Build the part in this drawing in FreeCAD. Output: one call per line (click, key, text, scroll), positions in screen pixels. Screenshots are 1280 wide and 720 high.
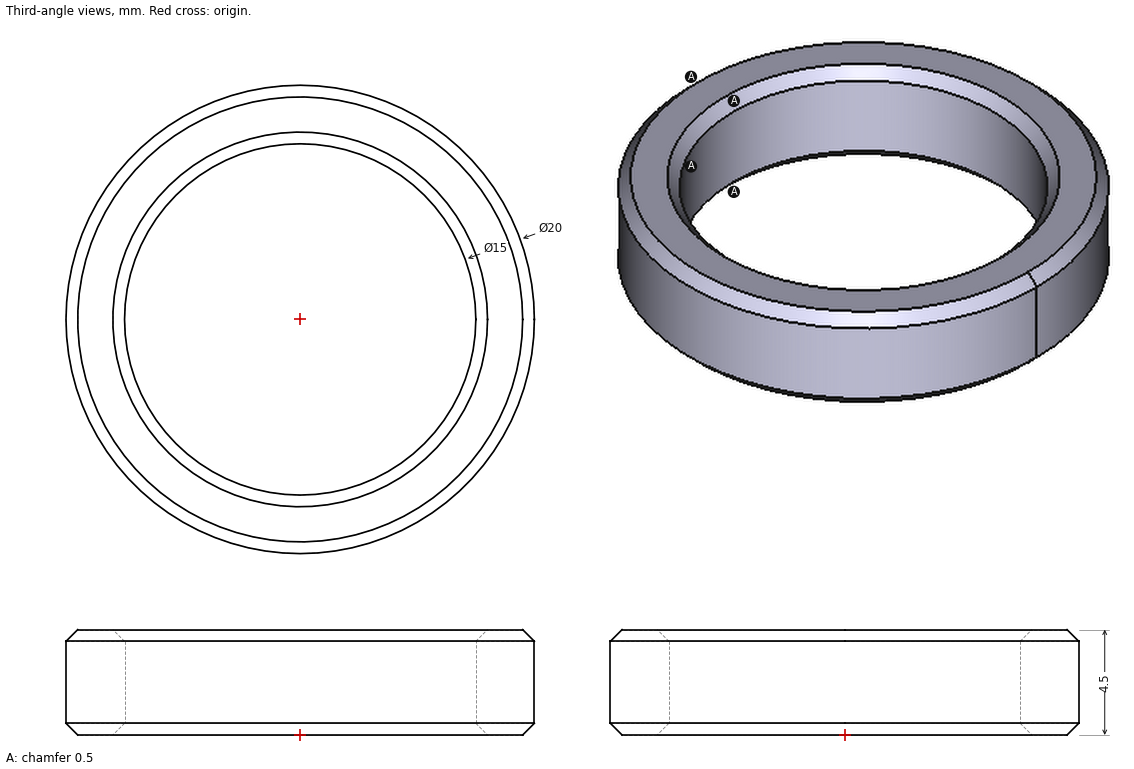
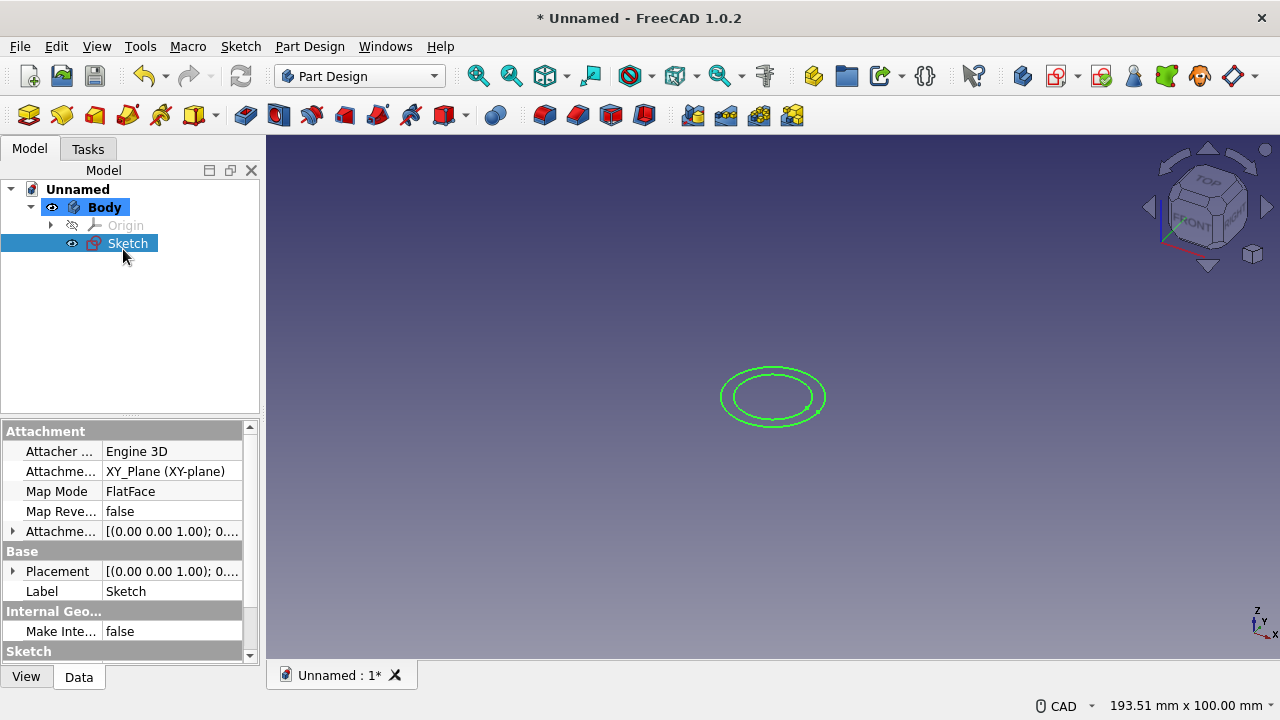
click(29, 116)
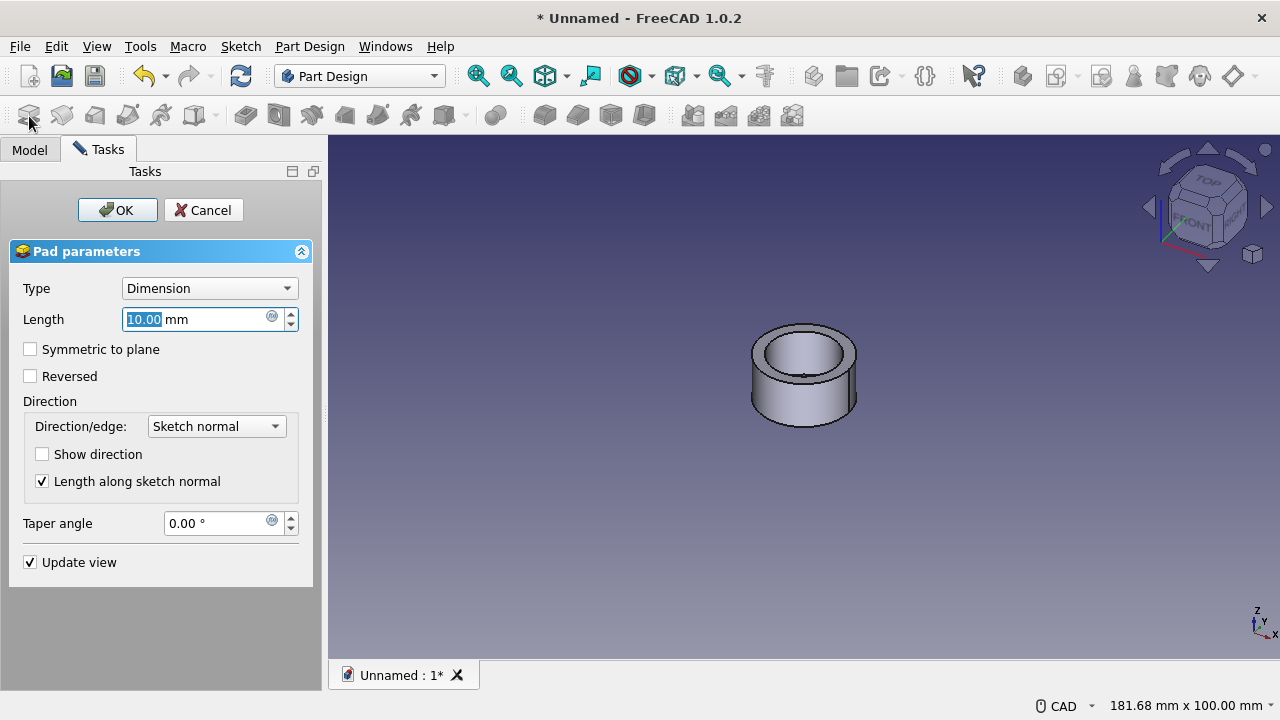
text(4.5)
key(Tab)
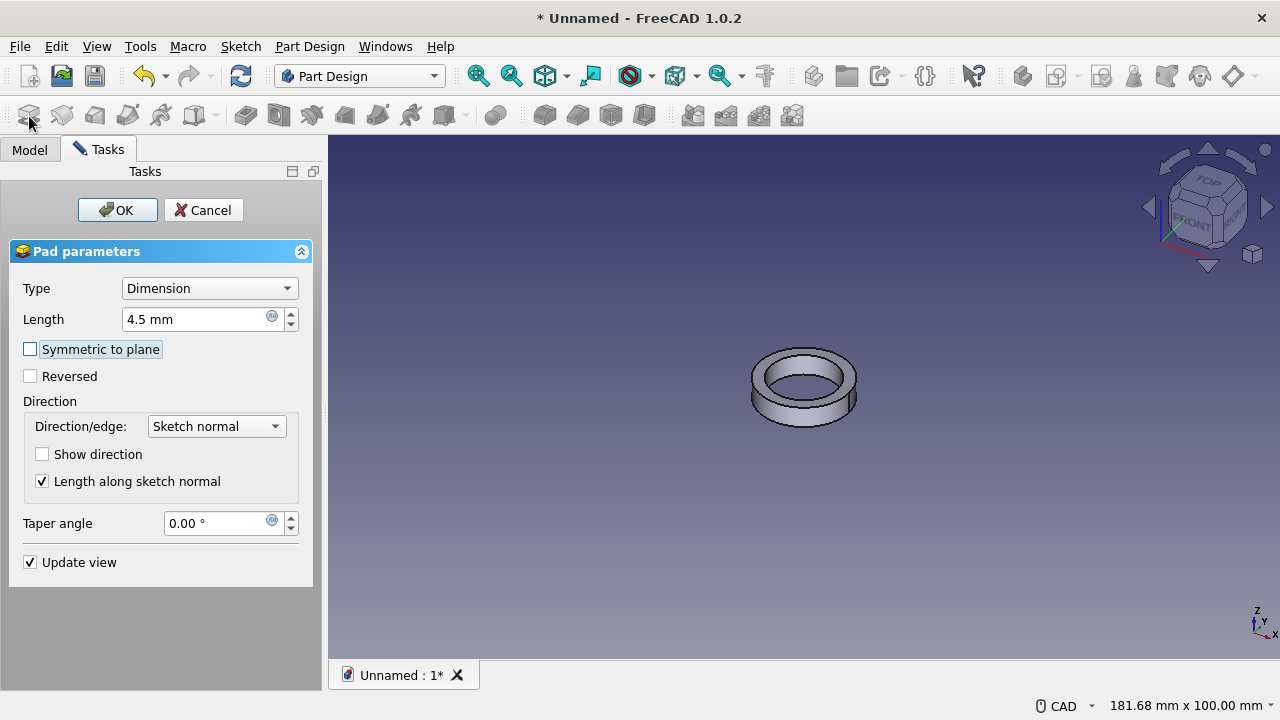
click(118, 210)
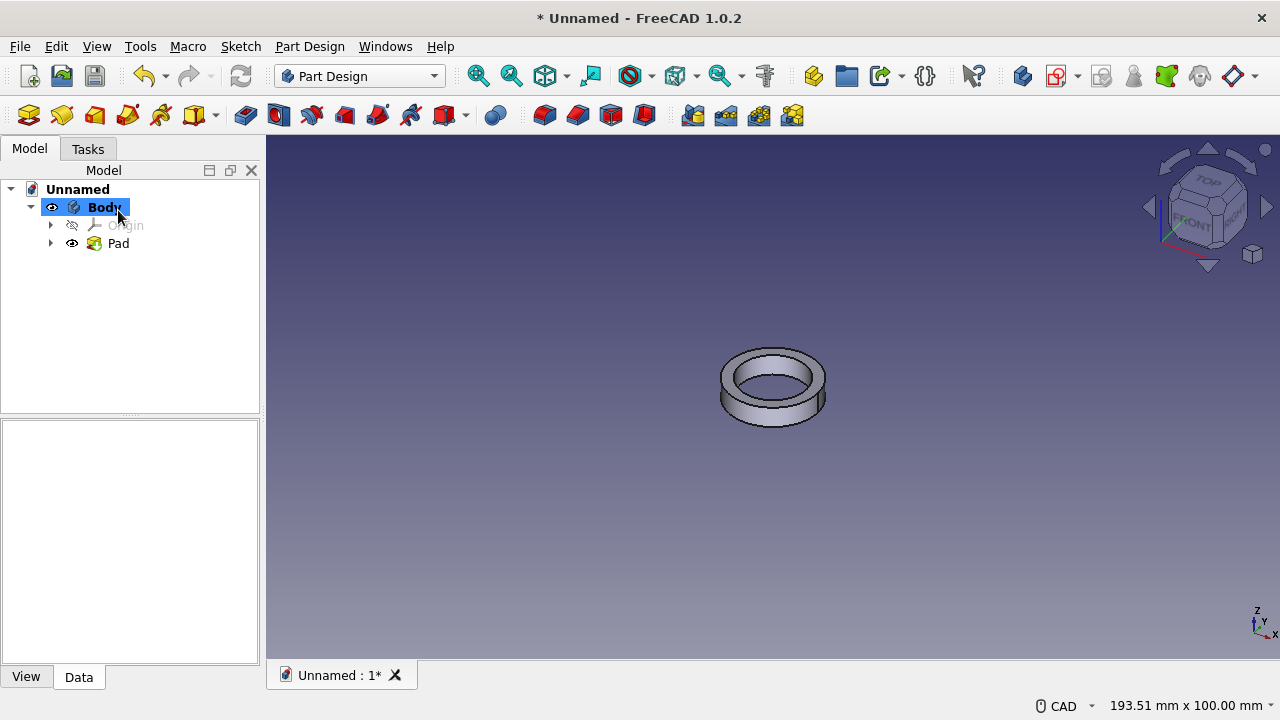
click(479, 76)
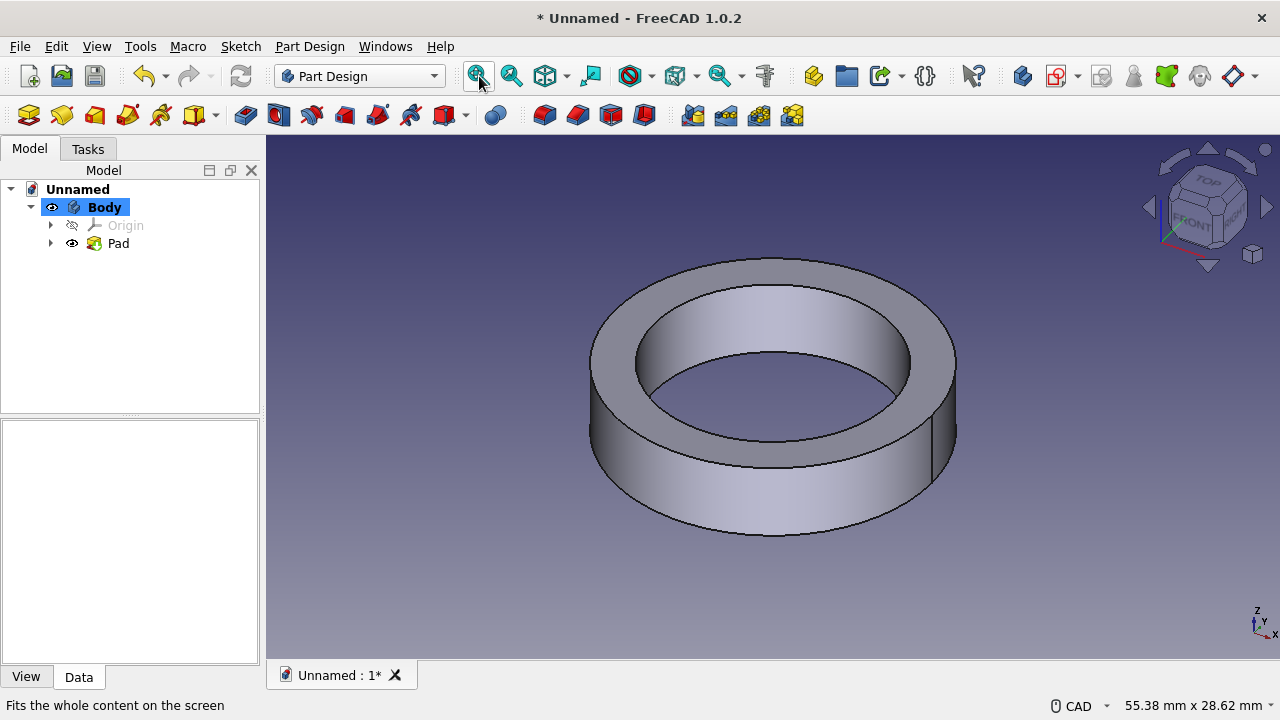
click(591, 373)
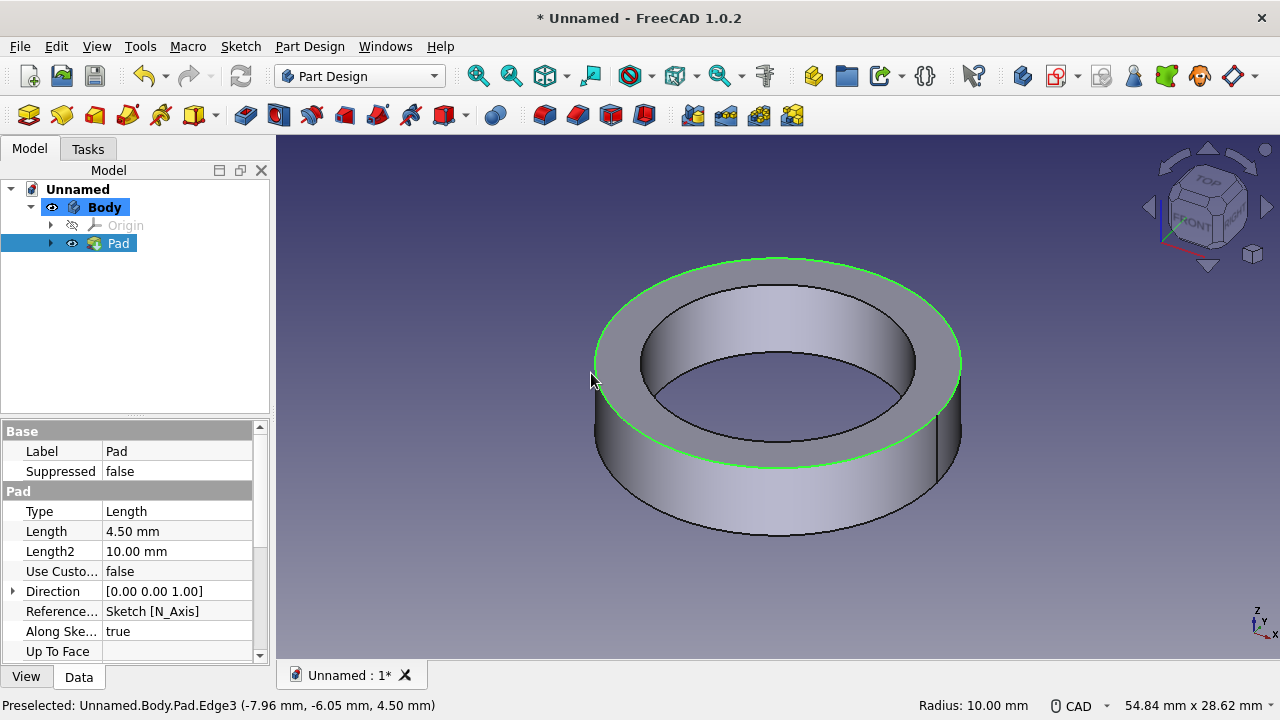
click(659, 323, ctrl)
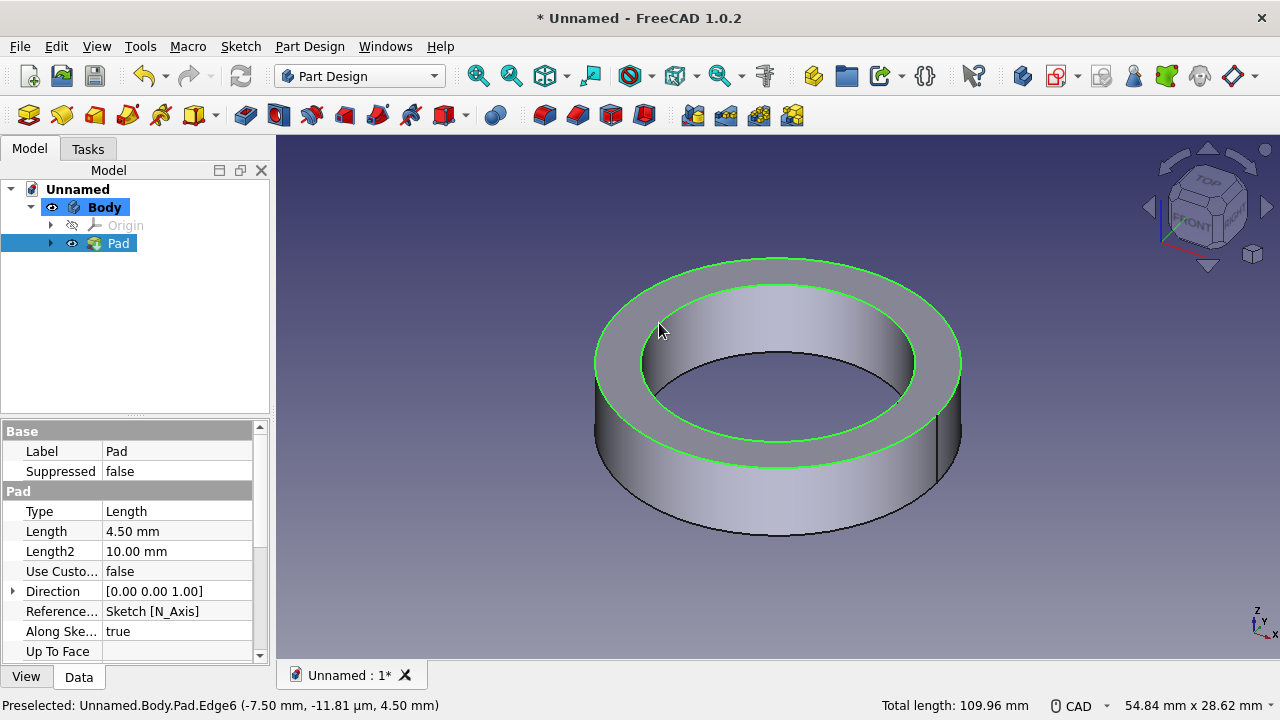
key(0)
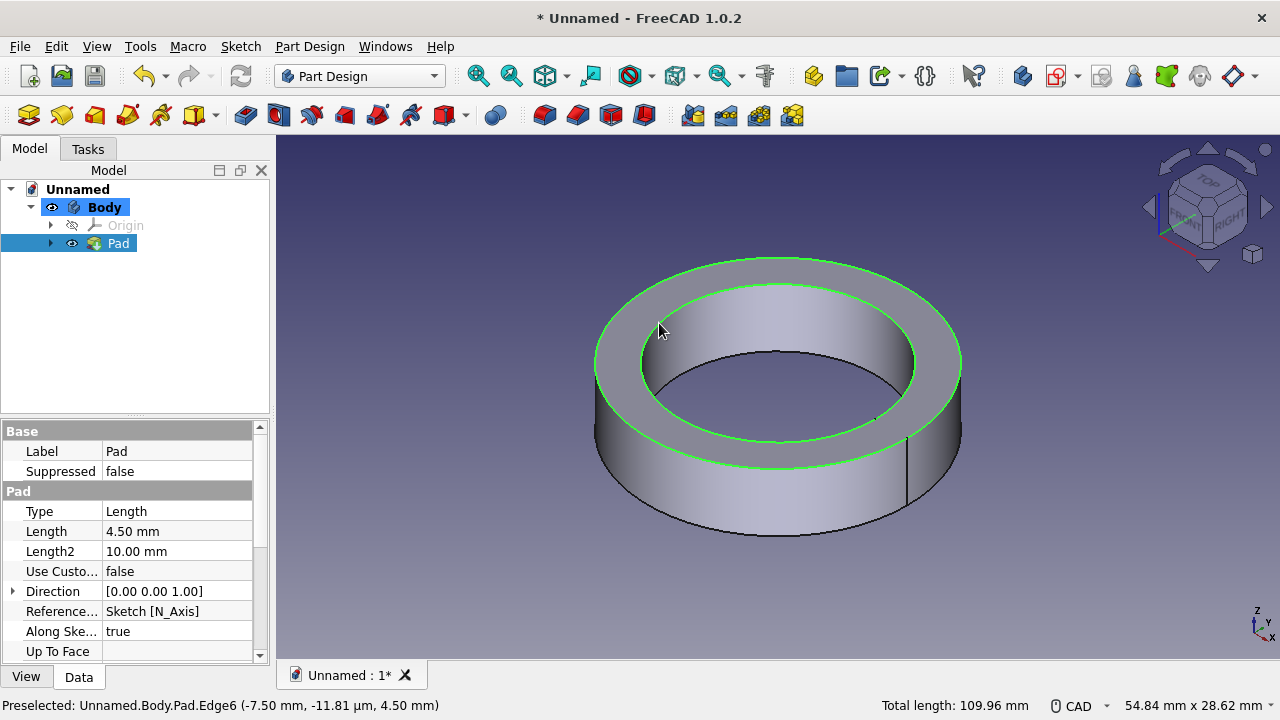
key(2)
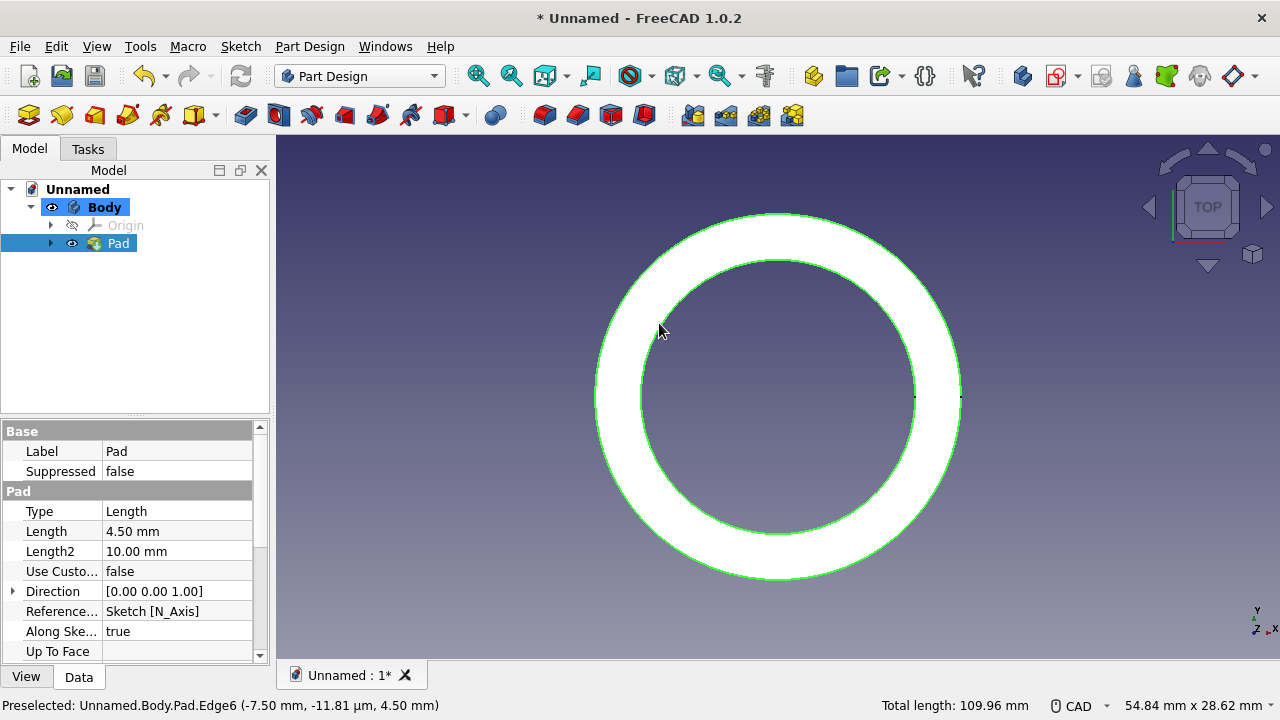
key(1)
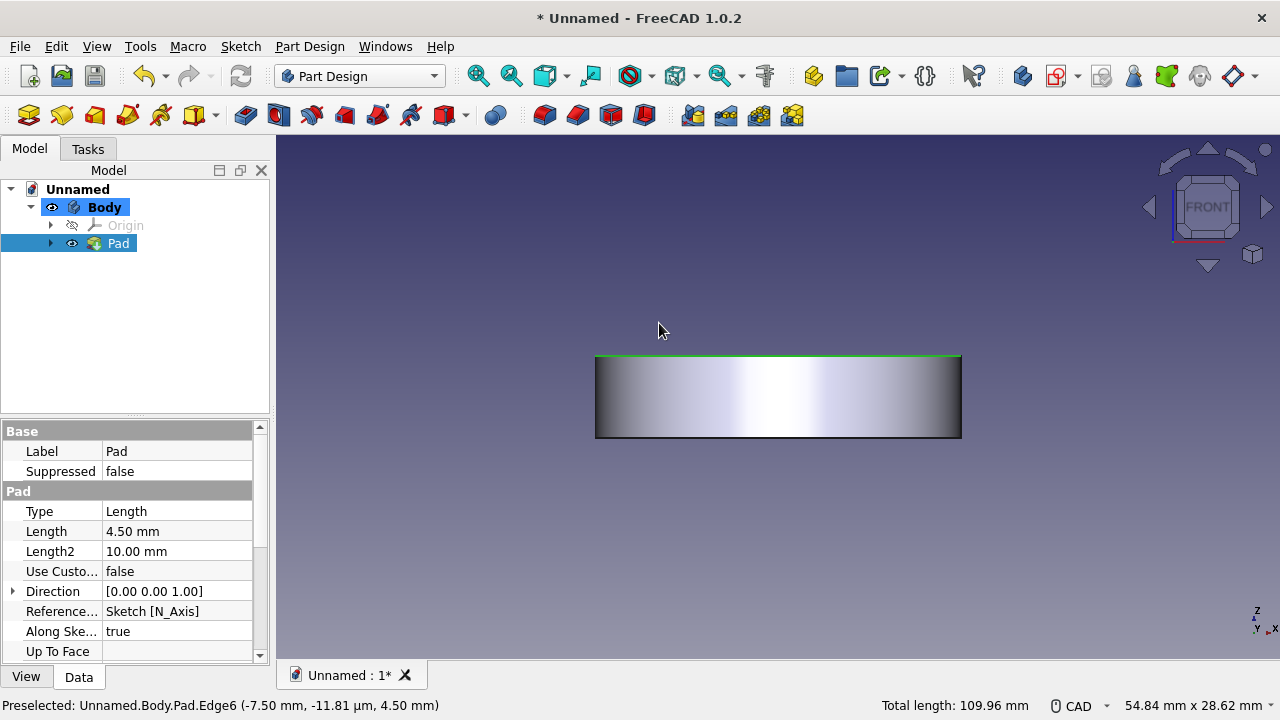
click(479, 76)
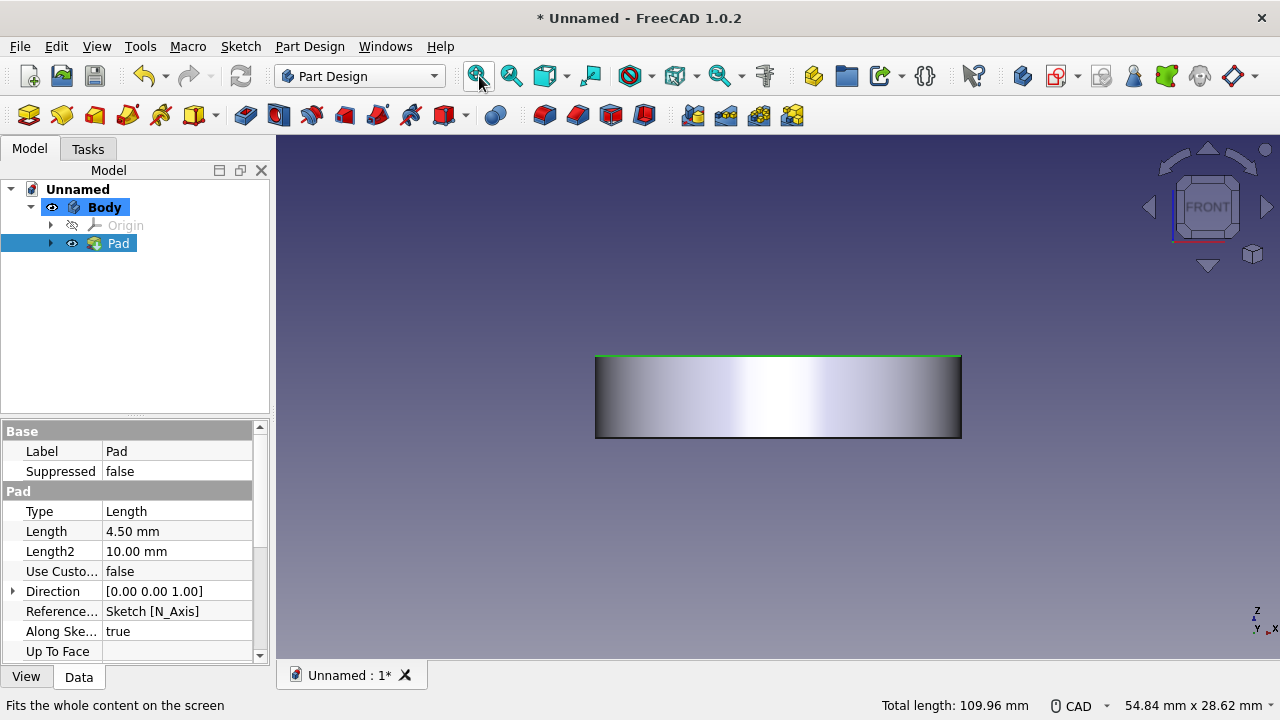
click(630, 437, ctrl)